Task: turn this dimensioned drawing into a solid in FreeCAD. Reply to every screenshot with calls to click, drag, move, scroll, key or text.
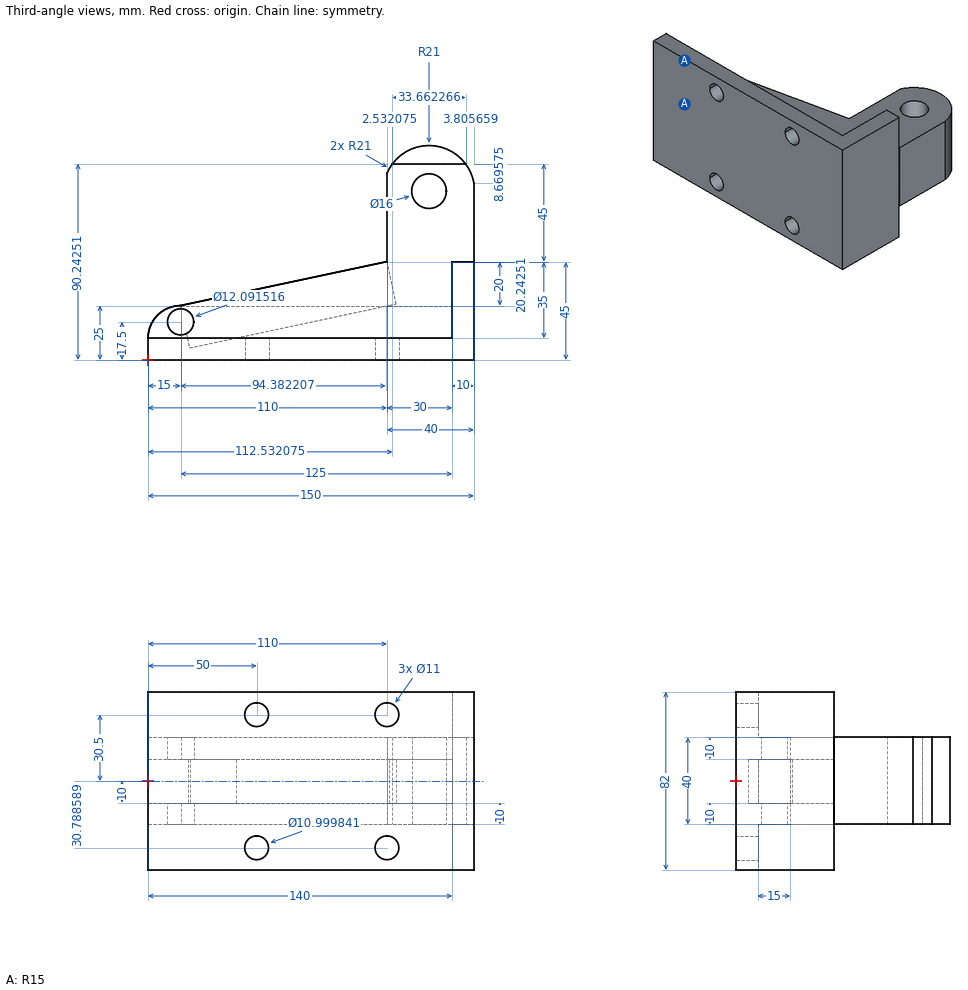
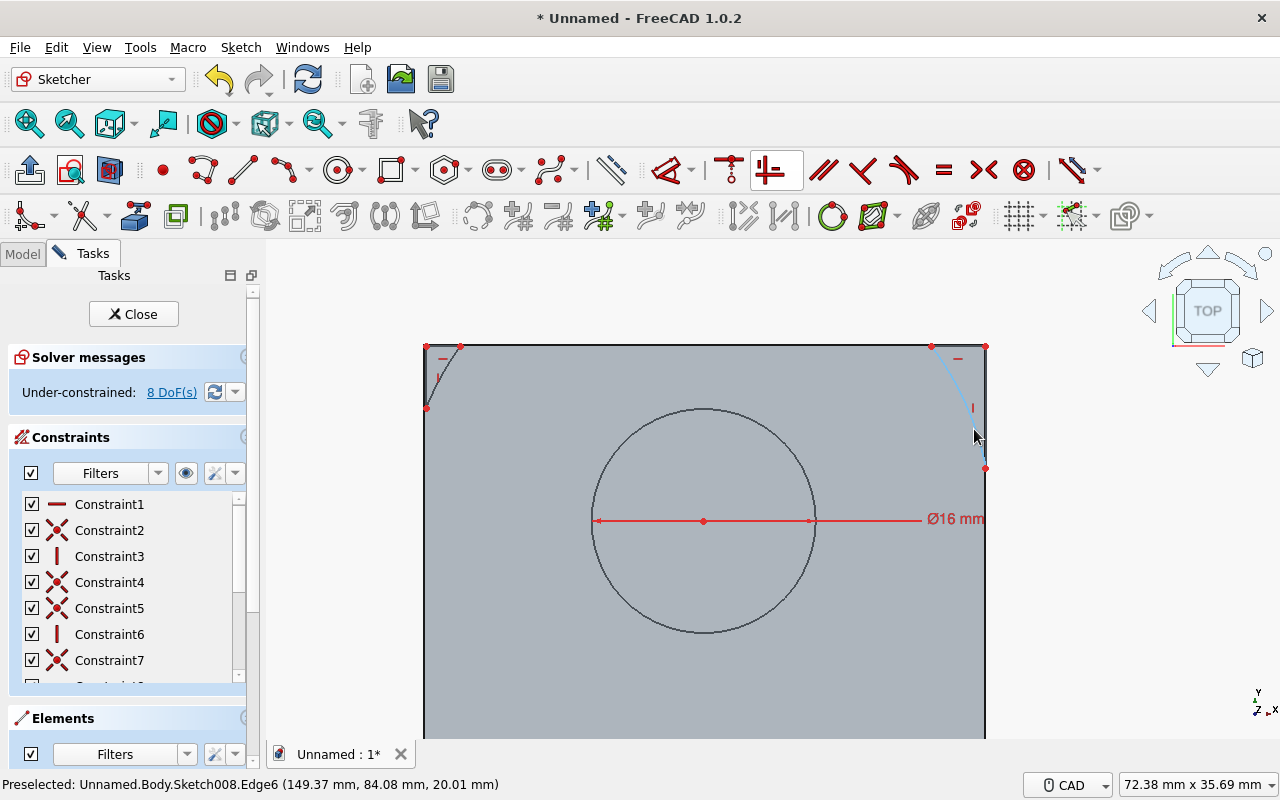
click(448, 364)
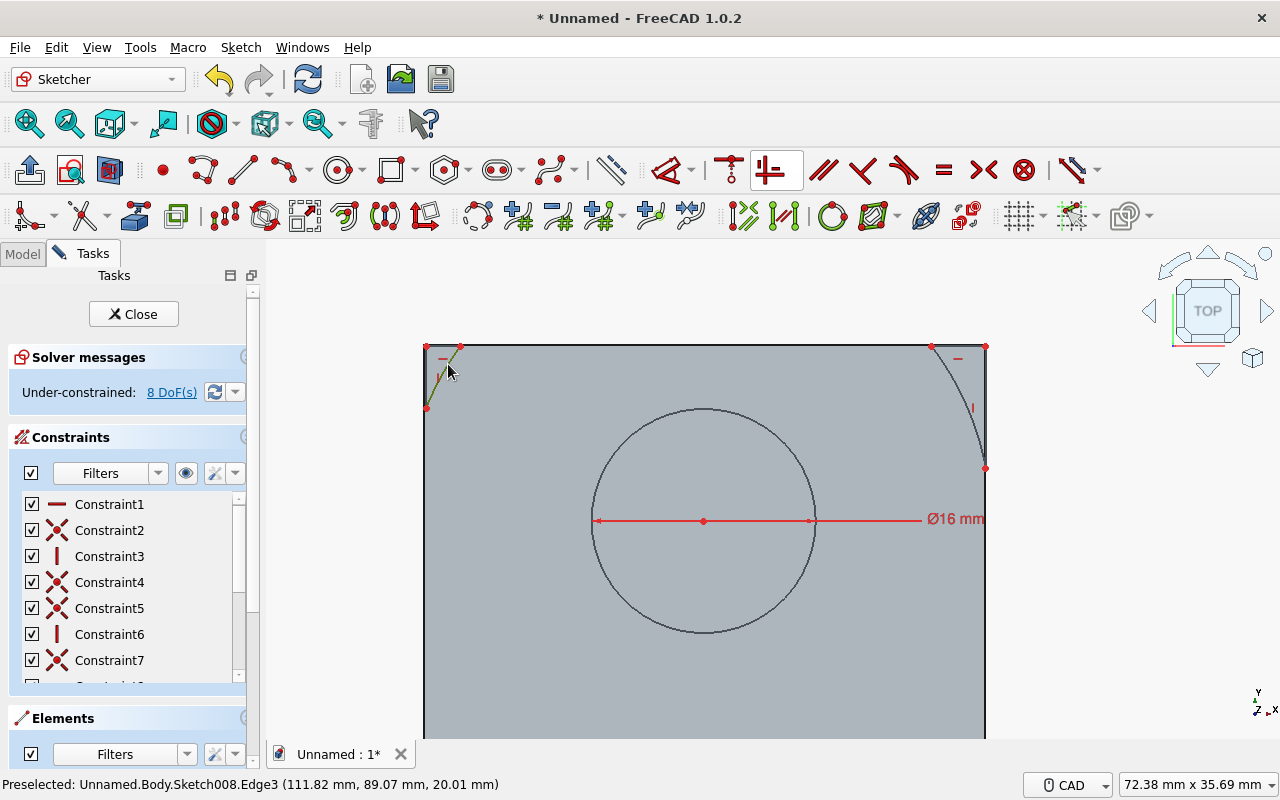
scroll(976, 429, up, 2)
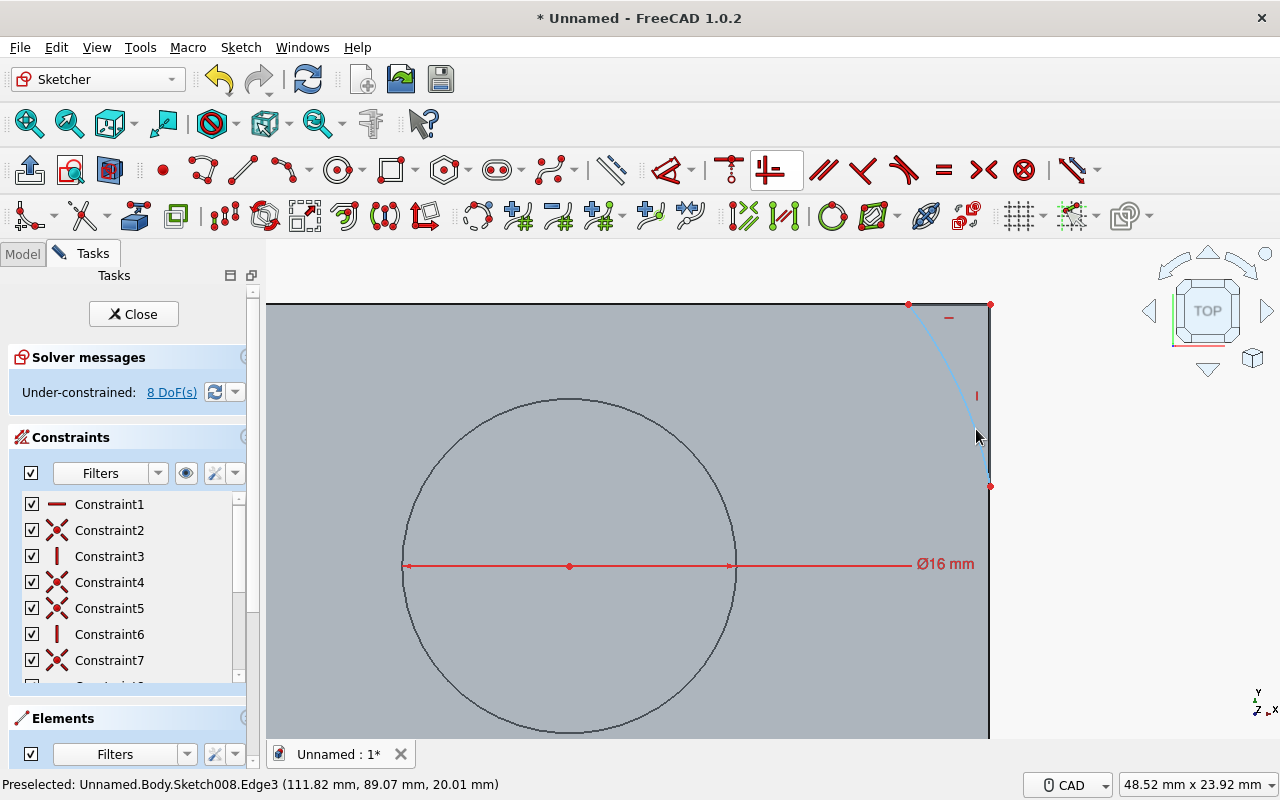
click(975, 429)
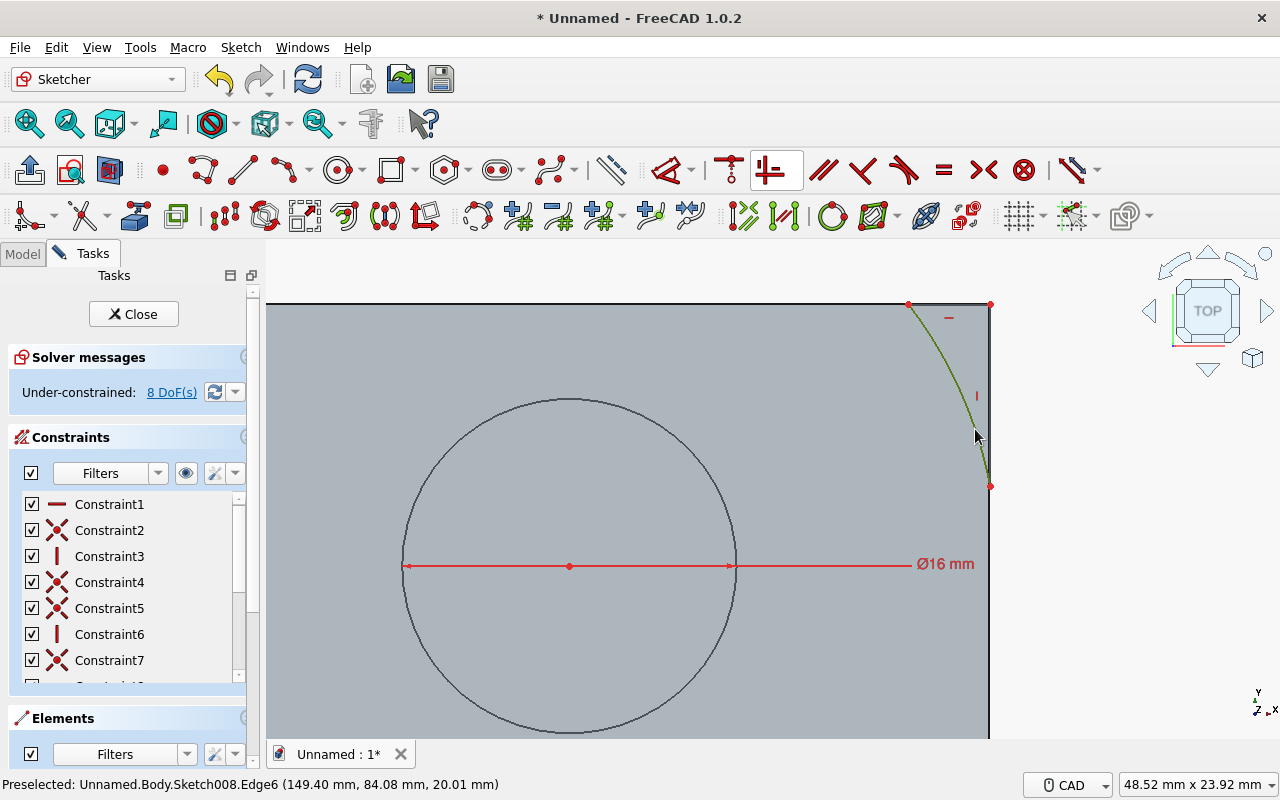
click(944, 170)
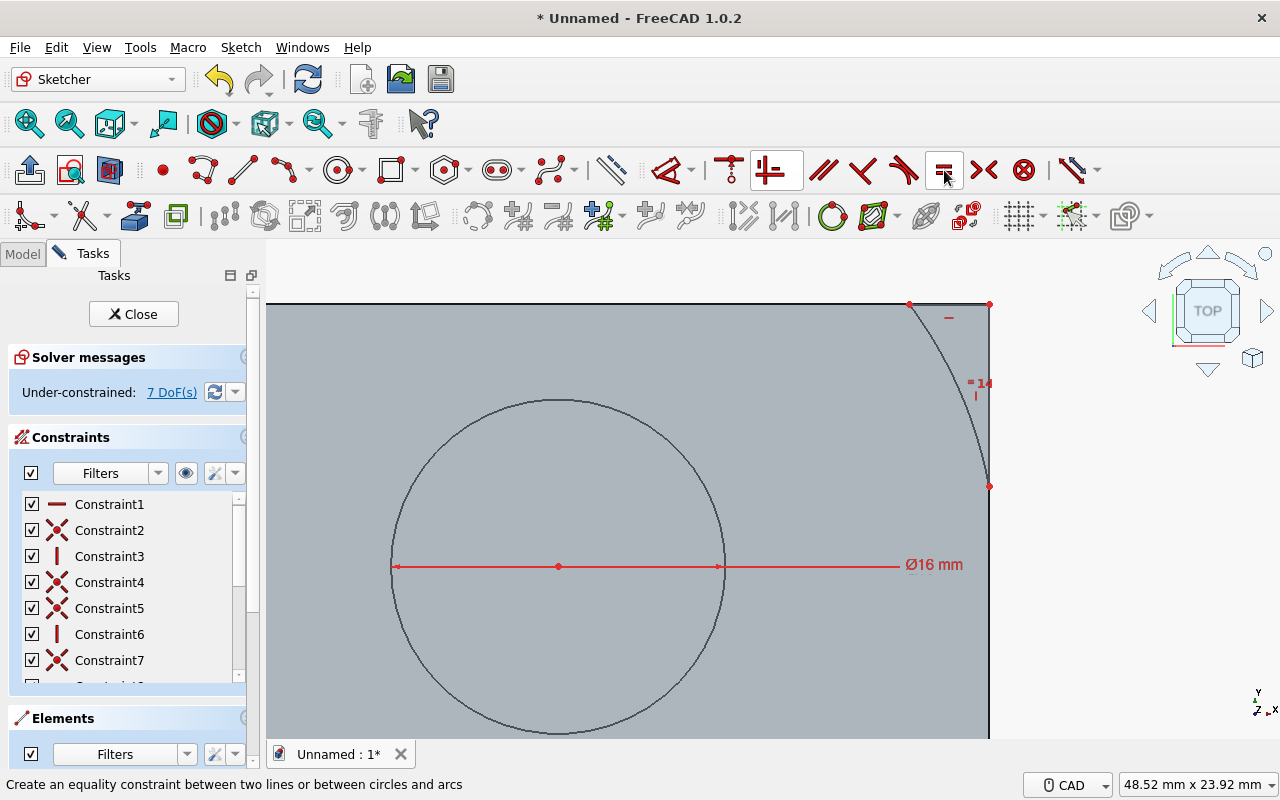
key(d)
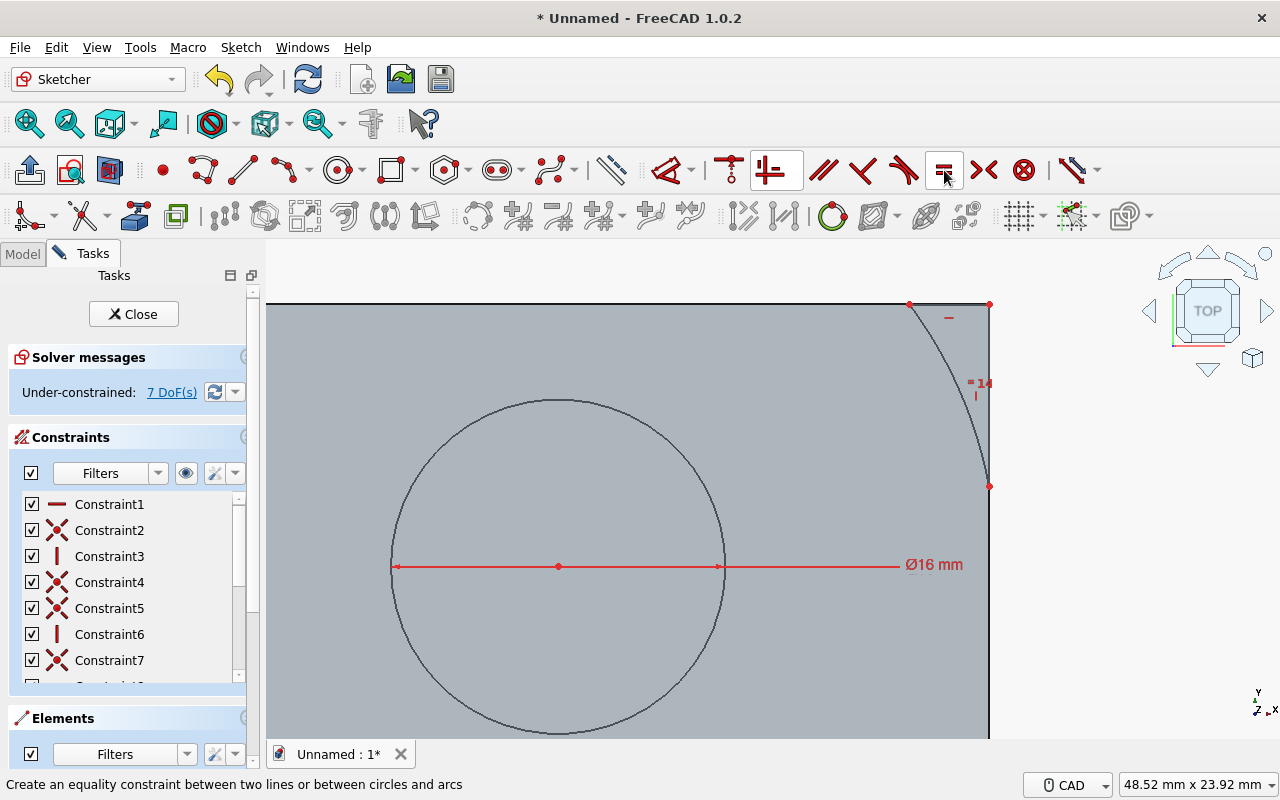
scroll(976, 429, down, 2)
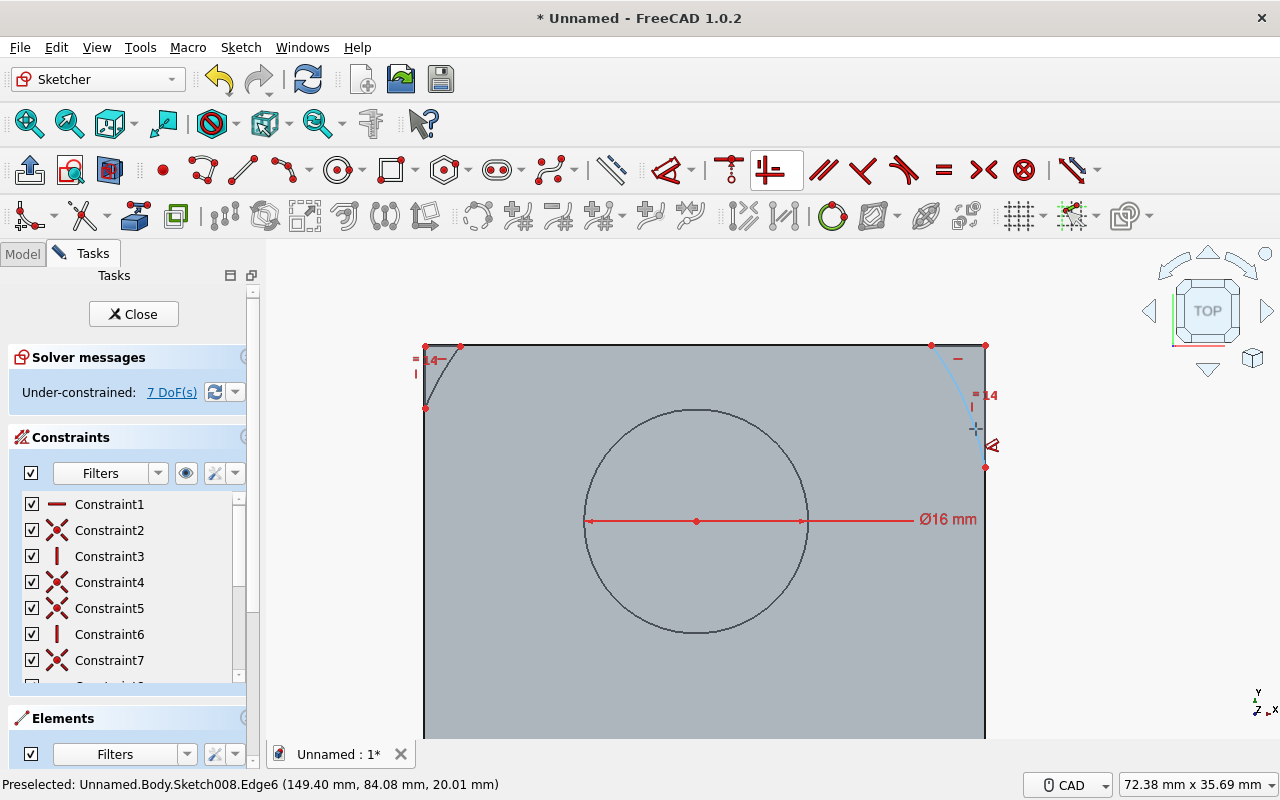
click(448, 364)
click(371, 500)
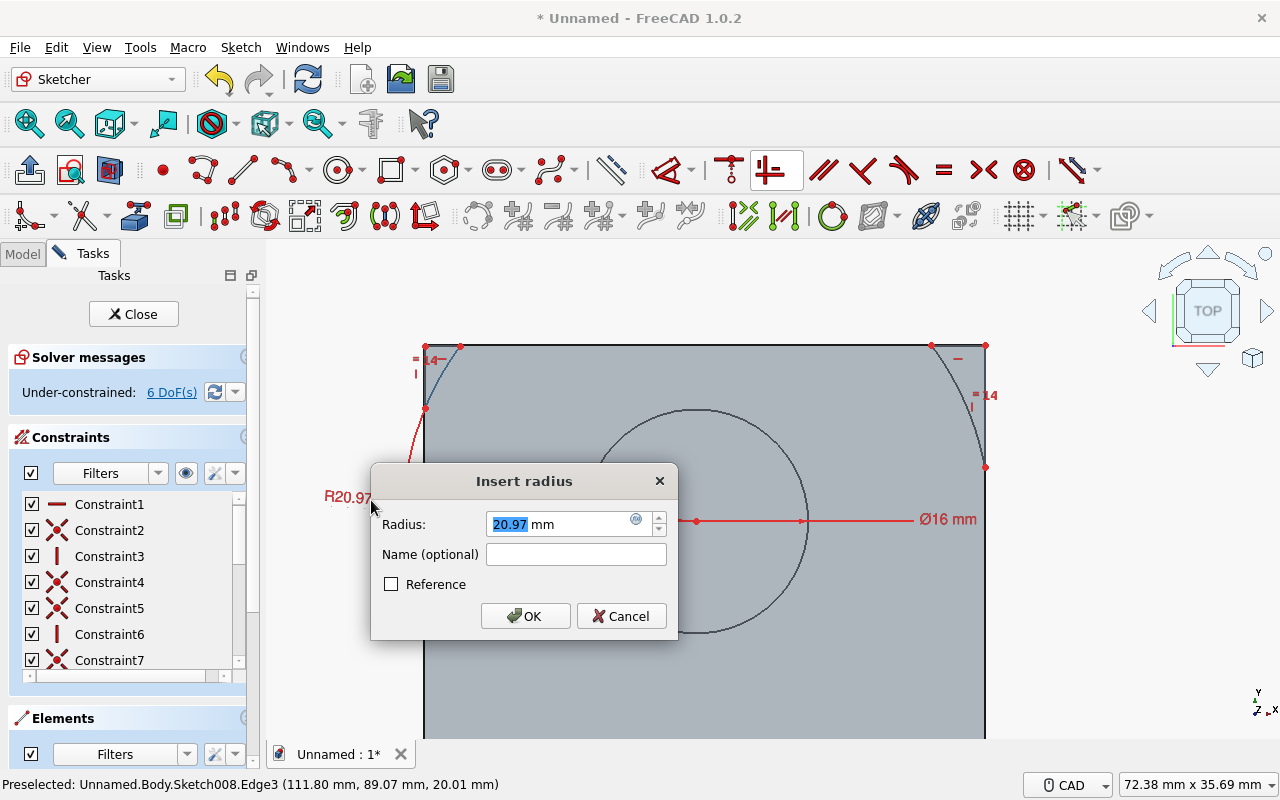
text(21)
key(Return)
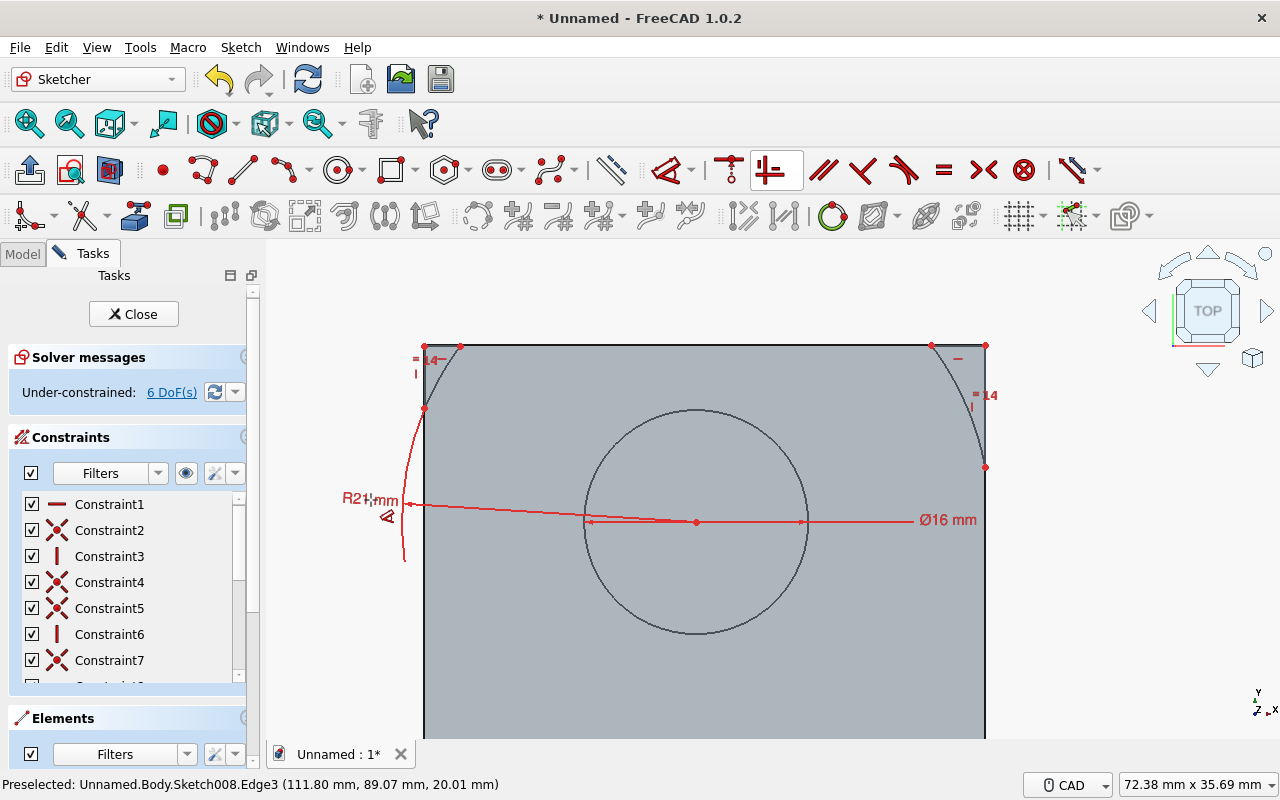
click(425, 346)
click(359, 312)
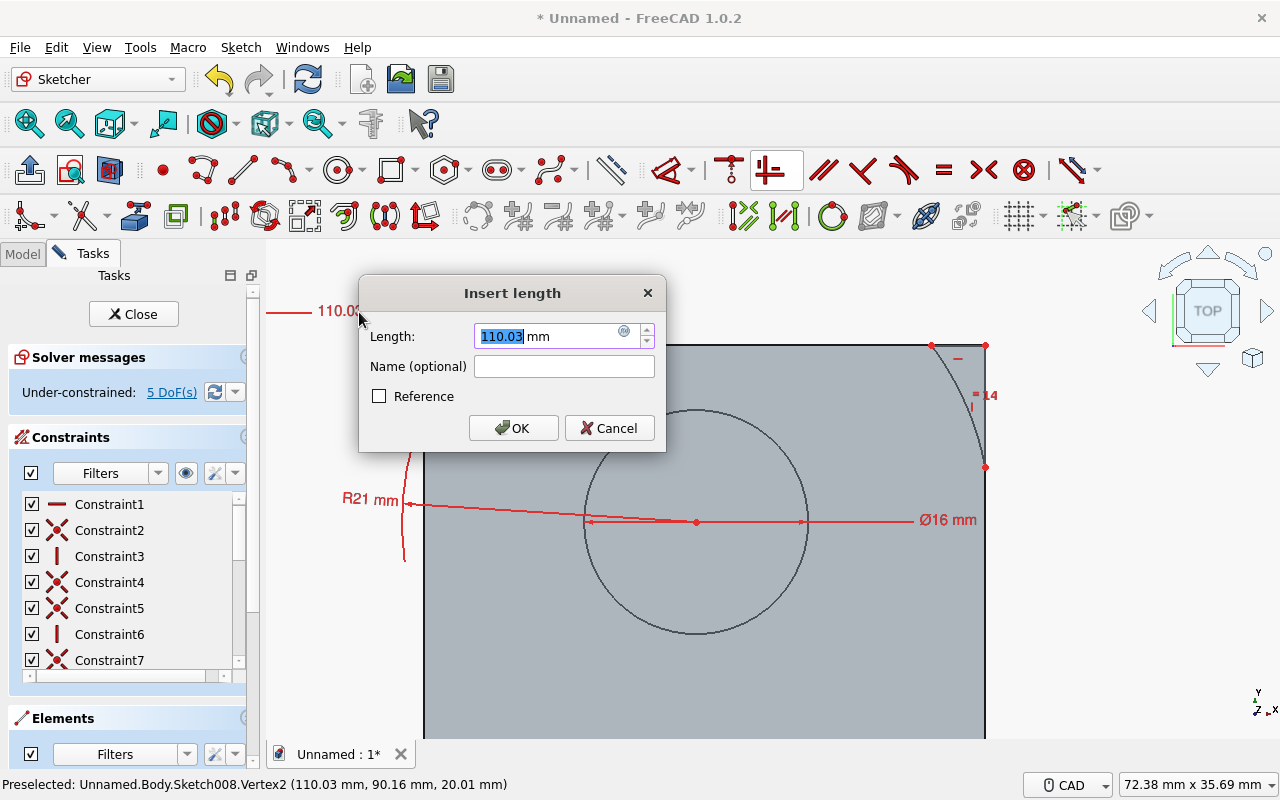
text(110)
key(Return)